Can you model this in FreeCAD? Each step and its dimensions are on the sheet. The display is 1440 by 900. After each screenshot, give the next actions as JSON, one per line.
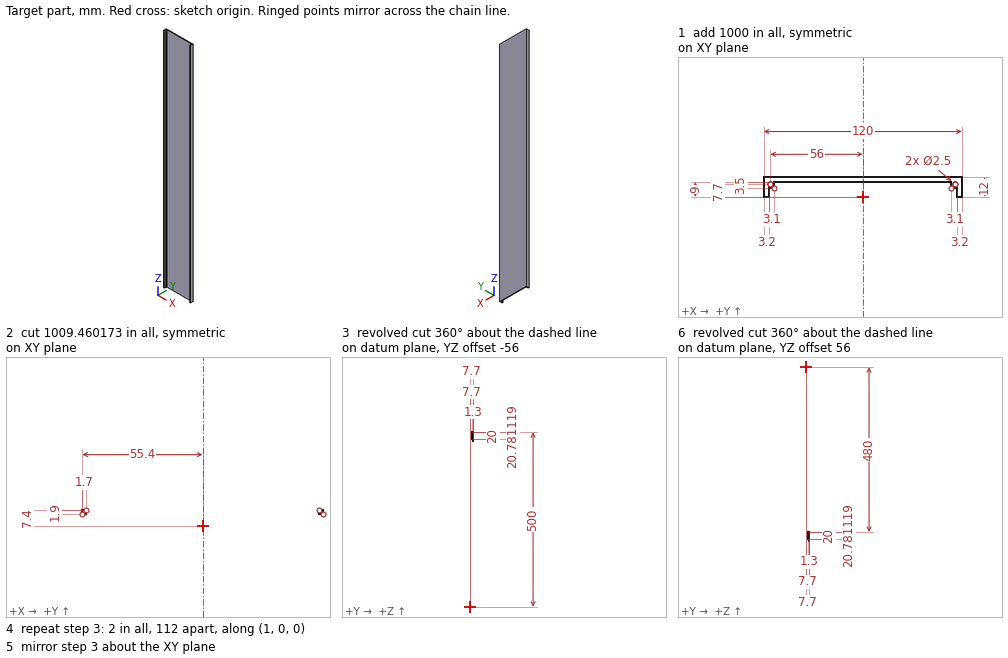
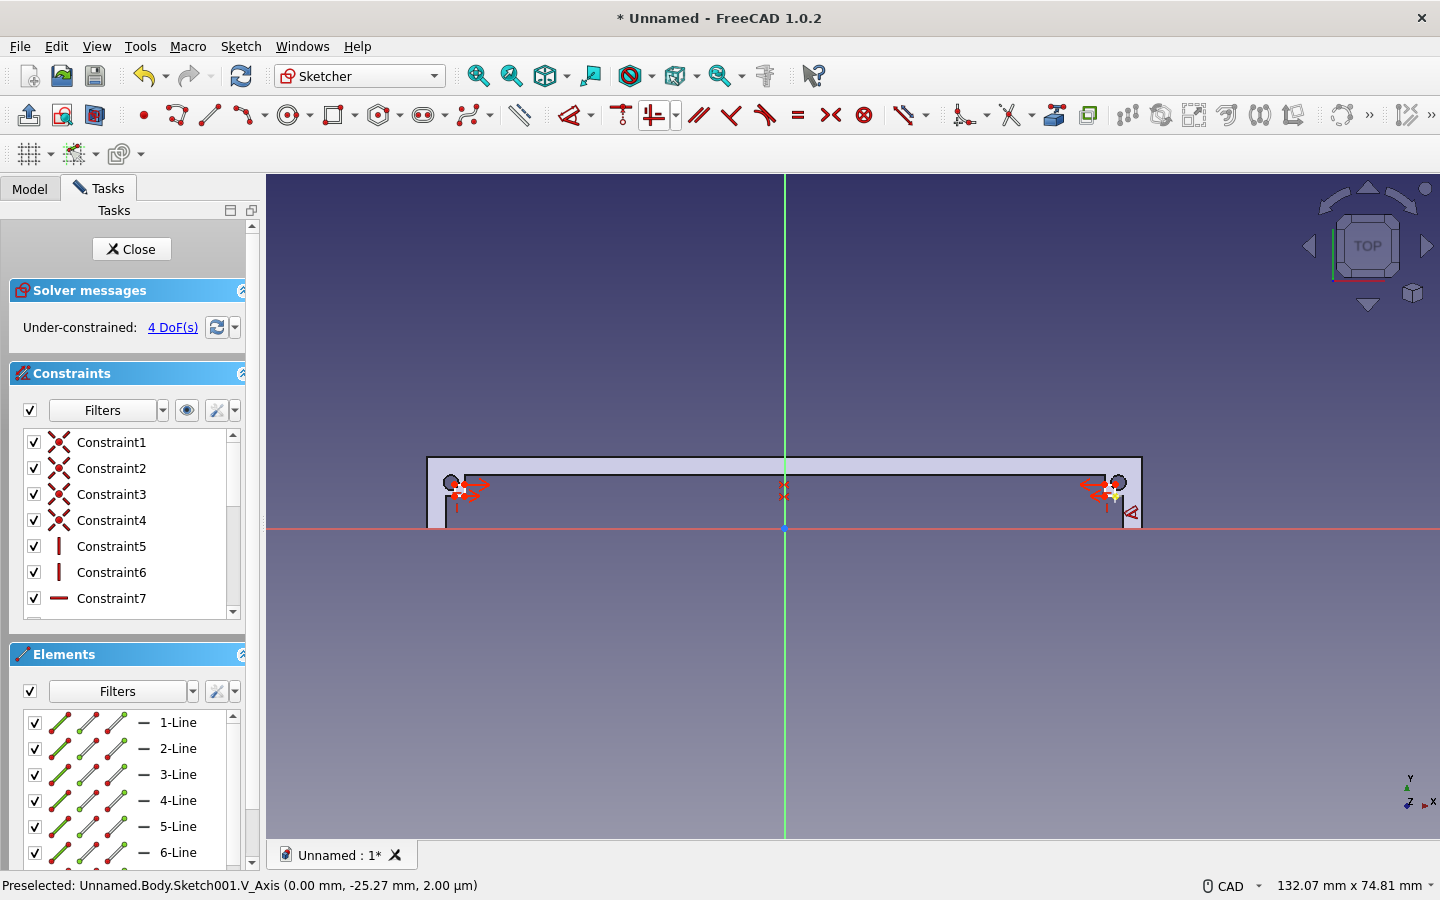
{"action": "scroll", "coordinate": [455, 490], "scroll_direction": "up", "scroll_amount": 7}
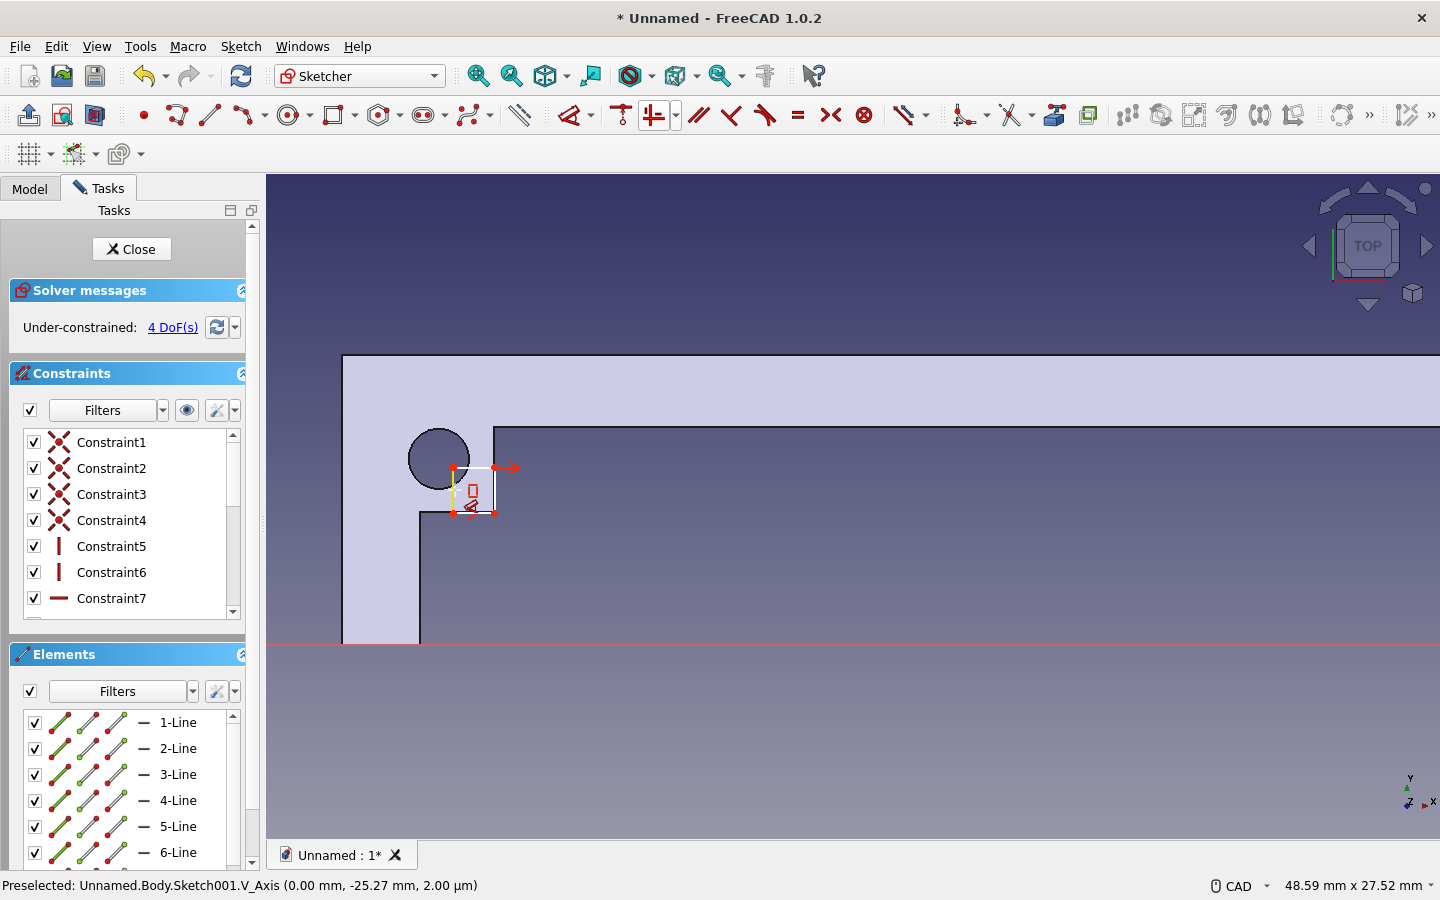
{"action": "left_click", "coordinate": [453, 491]}
{"action": "left_click", "coordinate": [419, 491]}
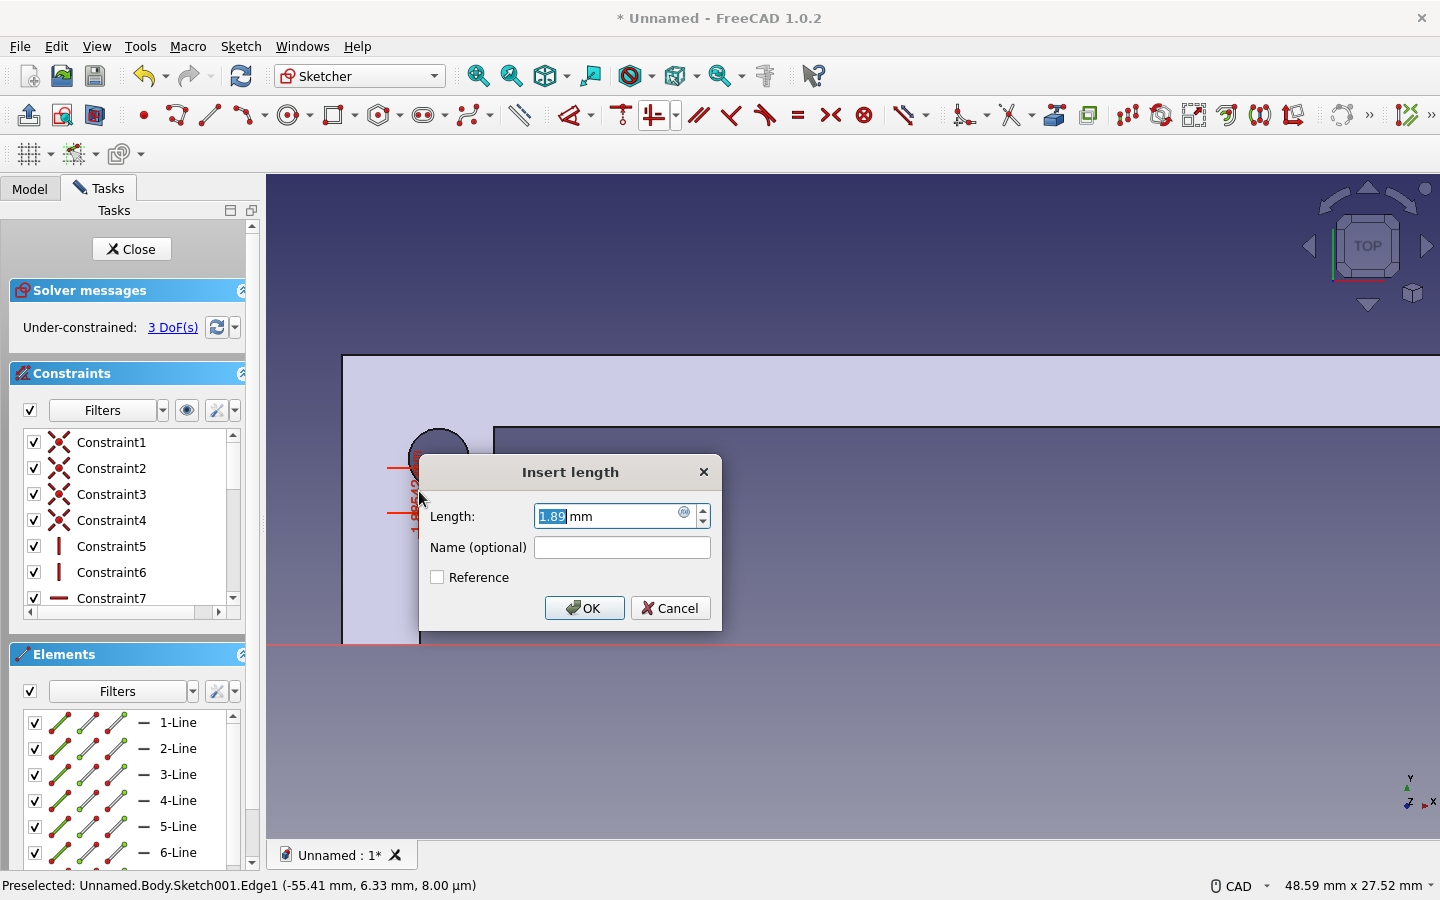
{"action": "type", "text": "1.9"}
{"action": "key", "text": "Return"}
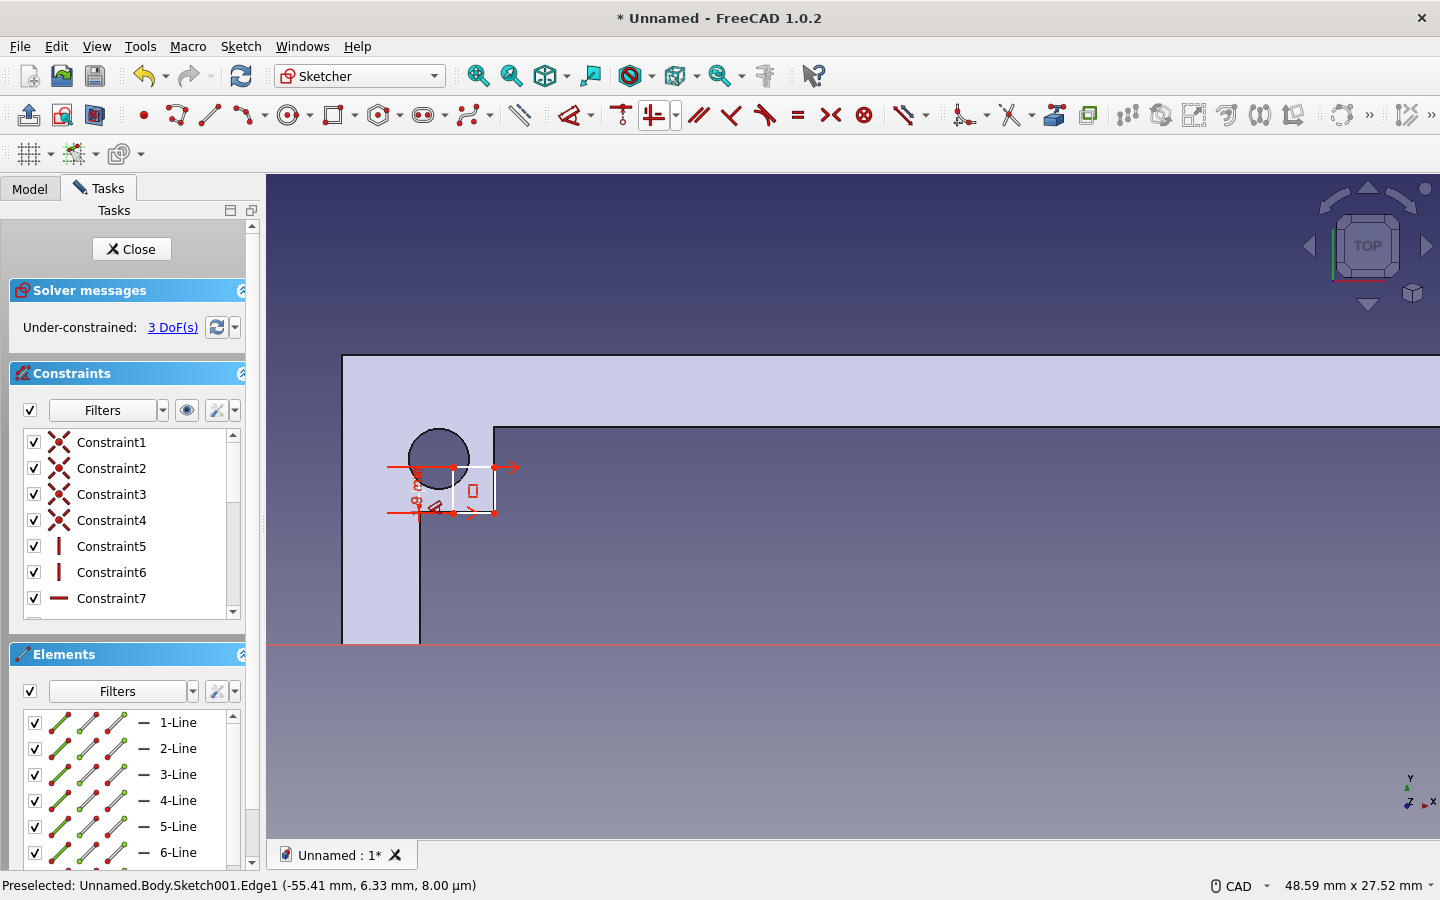
{"action": "left_click", "coordinate": [466, 513]}
{"action": "left_click", "coordinate": [474, 547]}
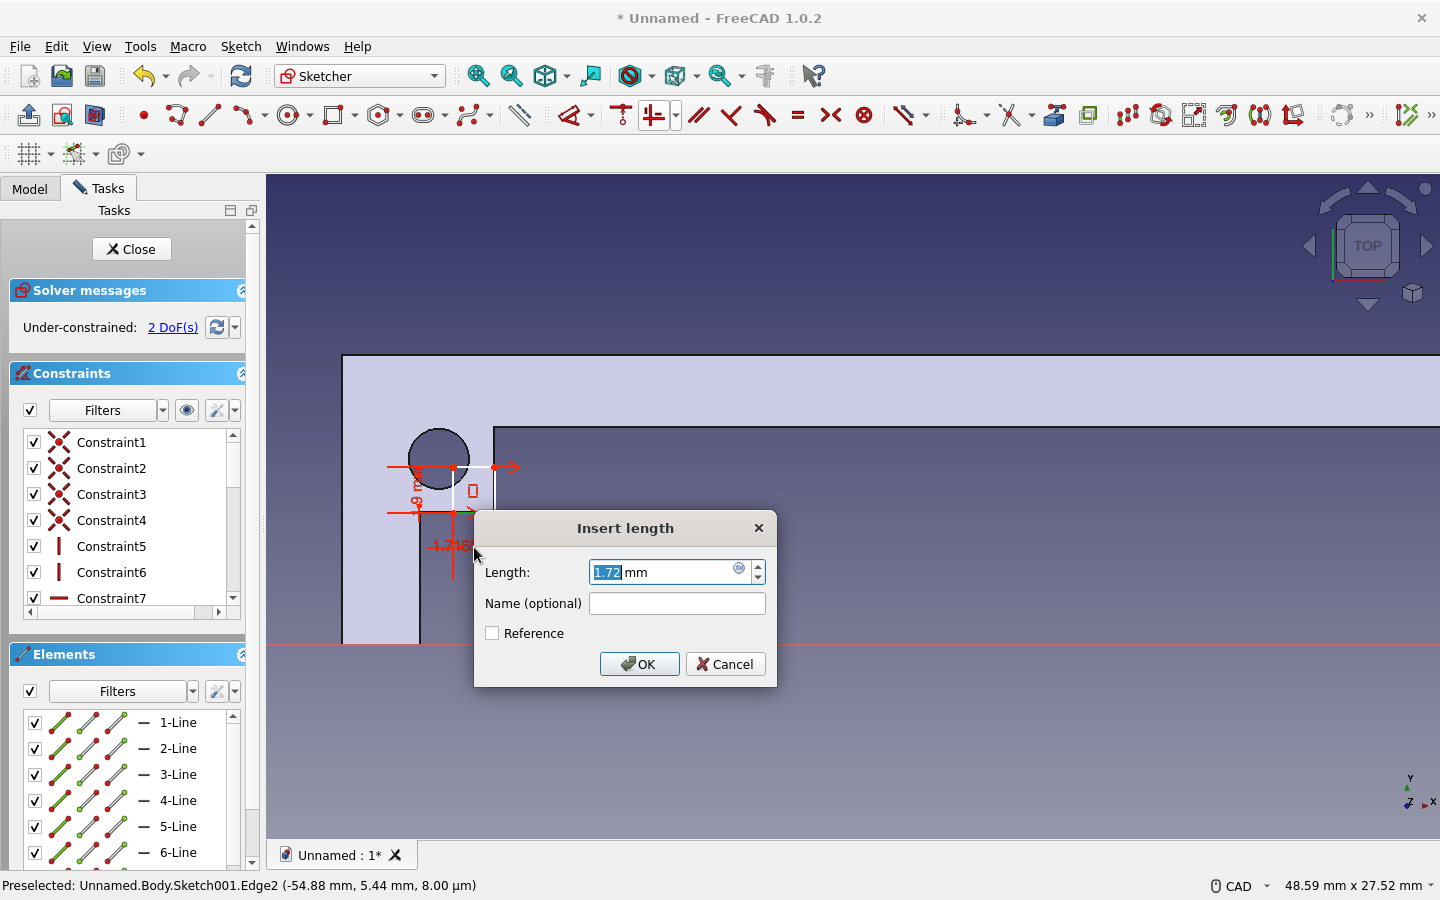
{"action": "type", "text": "1.7"}
{"action": "key", "text": "Return"}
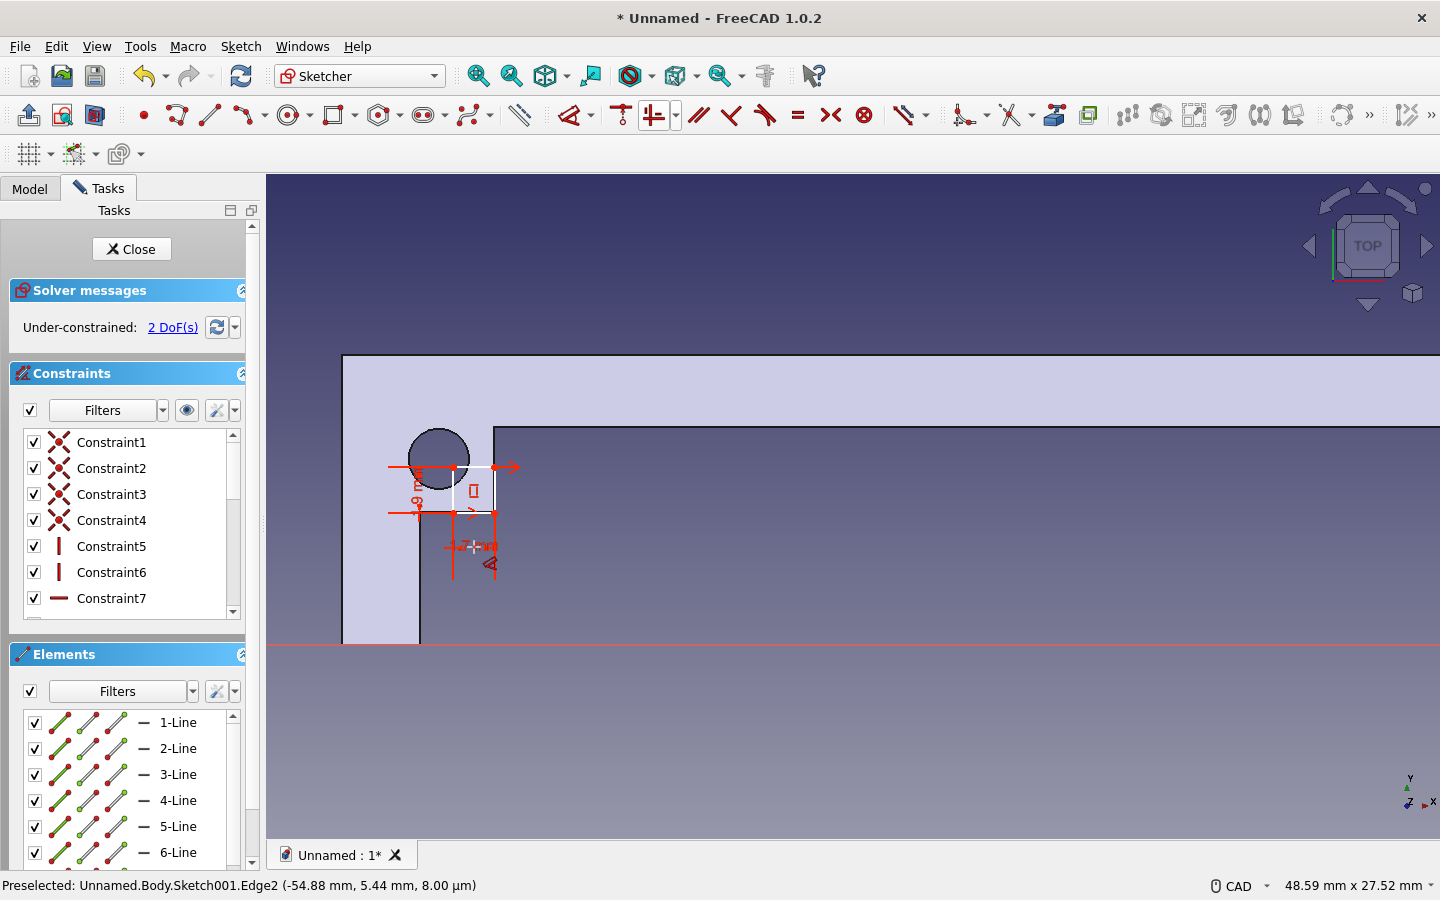
{"action": "scroll", "coordinate": [455, 490], "scroll_direction": "down", "scroll_amount": 7}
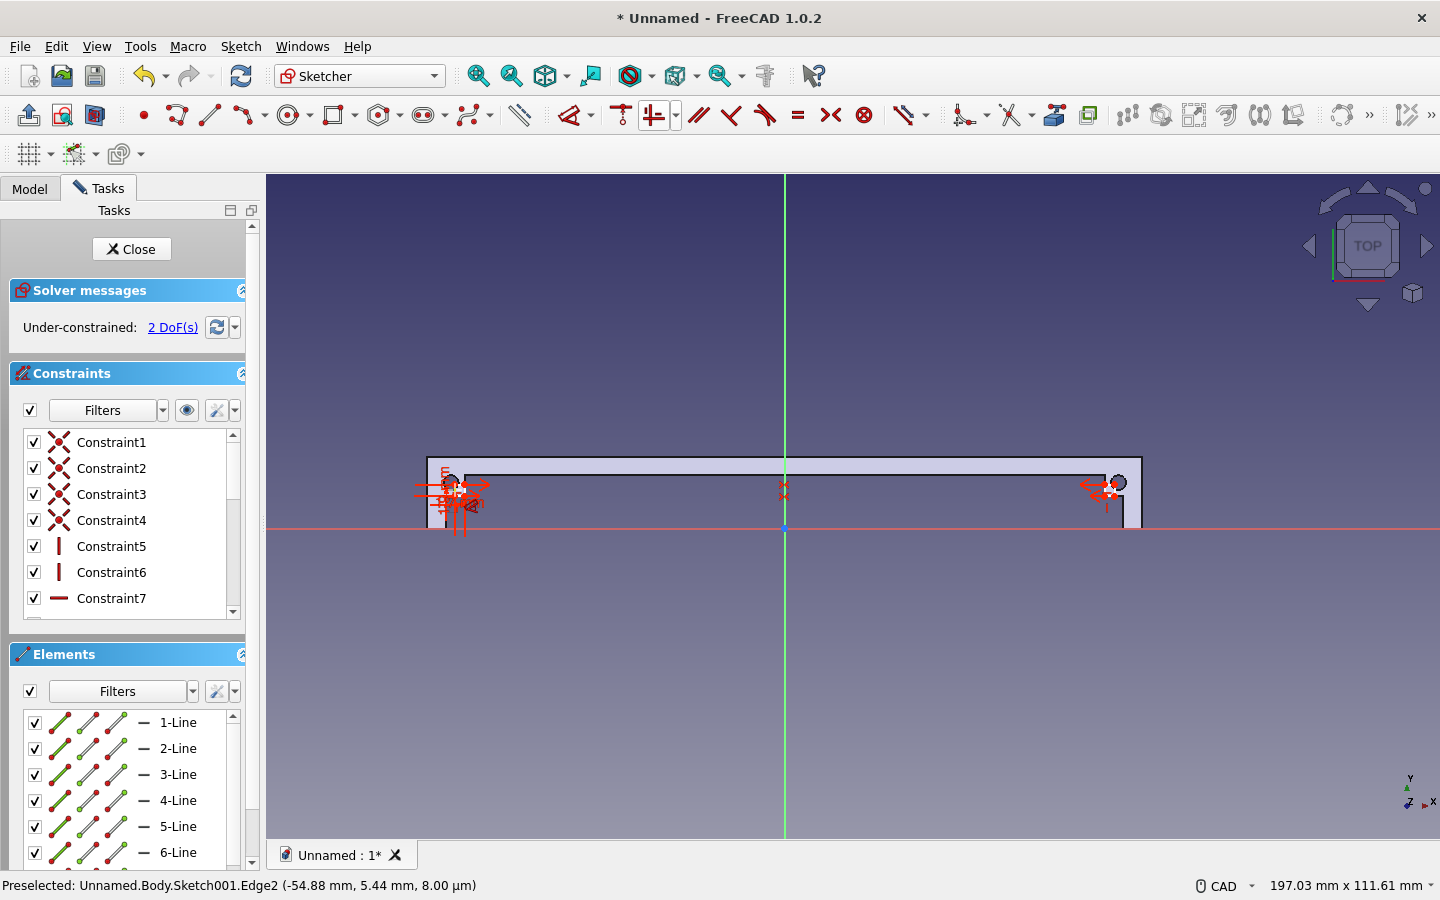
{"action": "left_click", "coordinate": [455, 485]}
{"action": "left_click", "coordinate": [819, 507]}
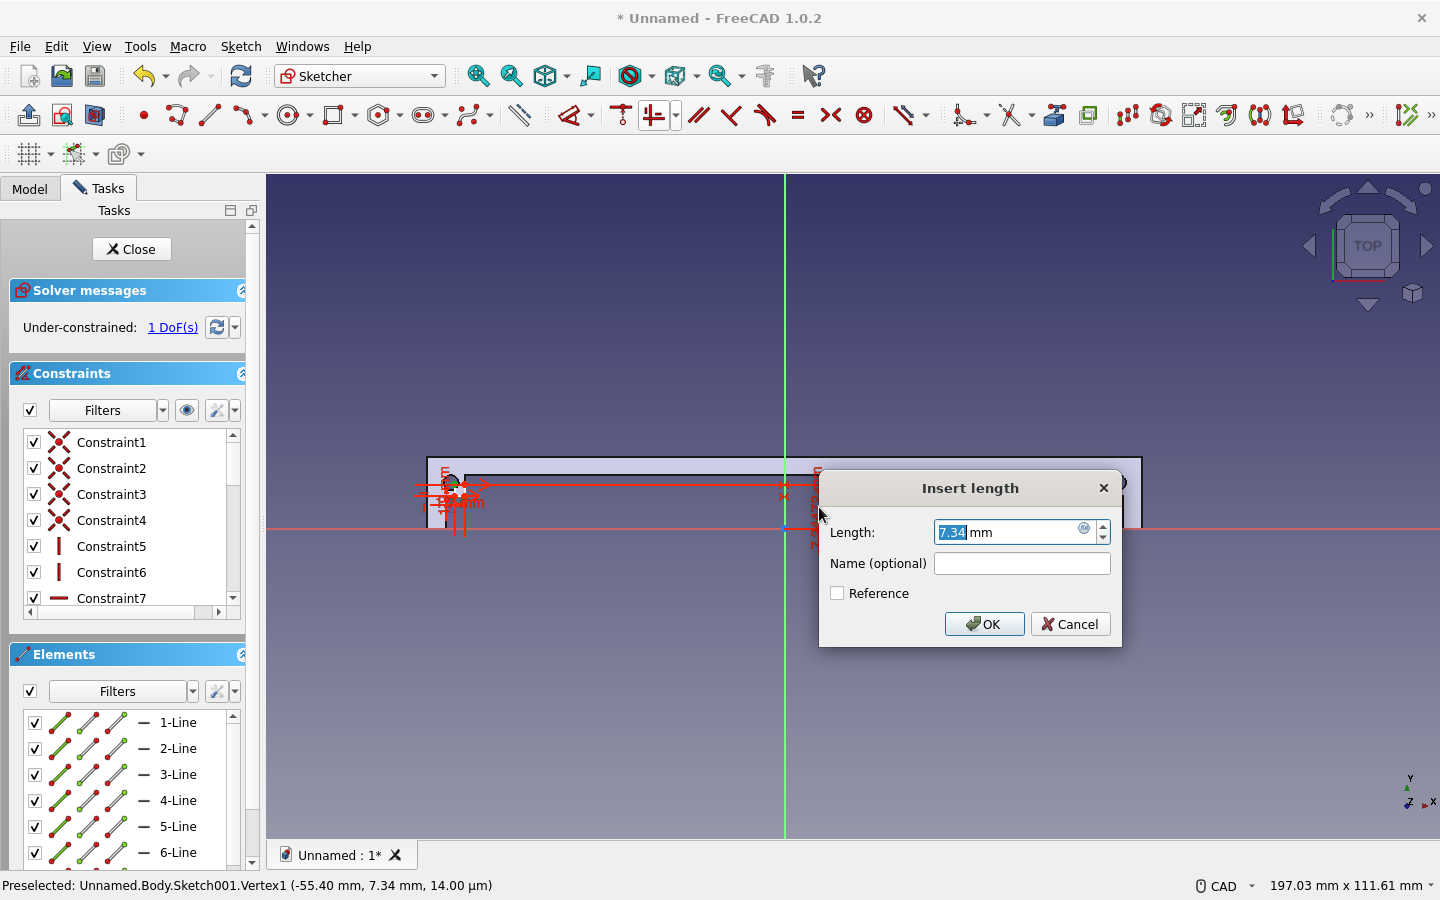
{"action": "type", "text": "7.4"}
{"action": "key", "text": "Return"}